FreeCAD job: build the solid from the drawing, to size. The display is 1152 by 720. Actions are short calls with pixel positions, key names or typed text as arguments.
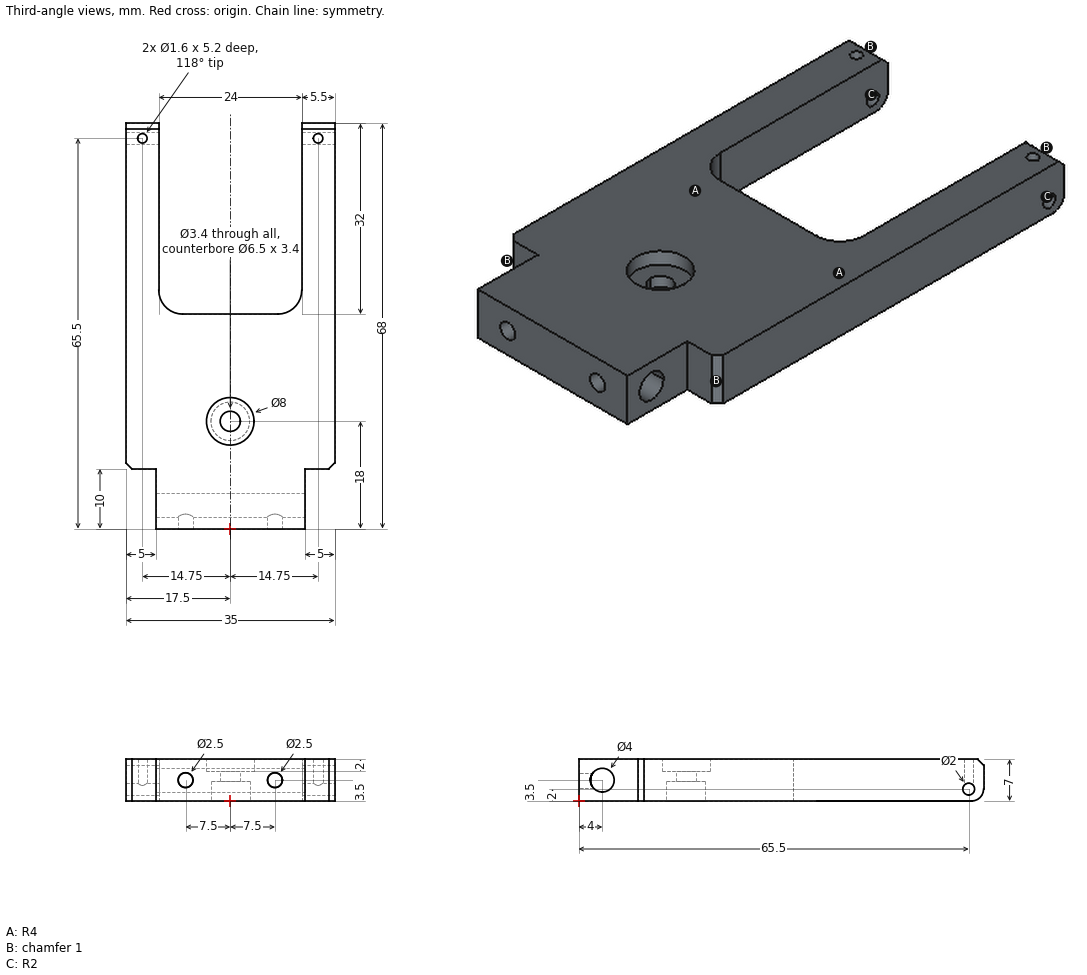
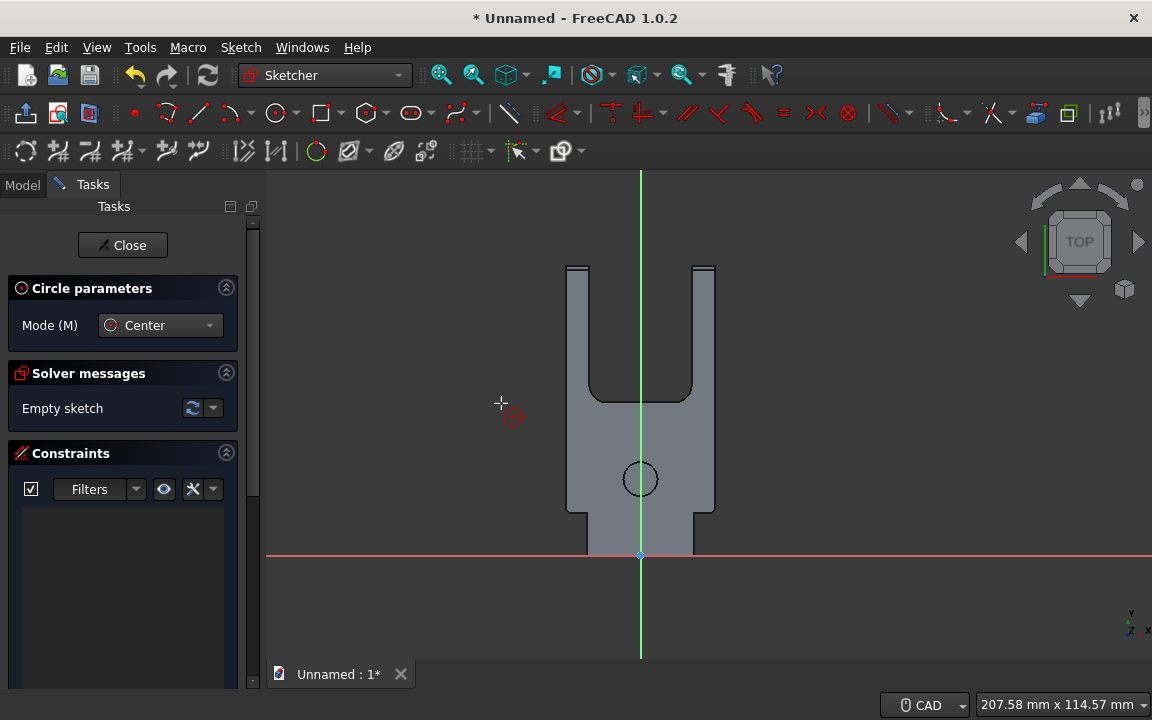
scroll(578, 276, up, 10)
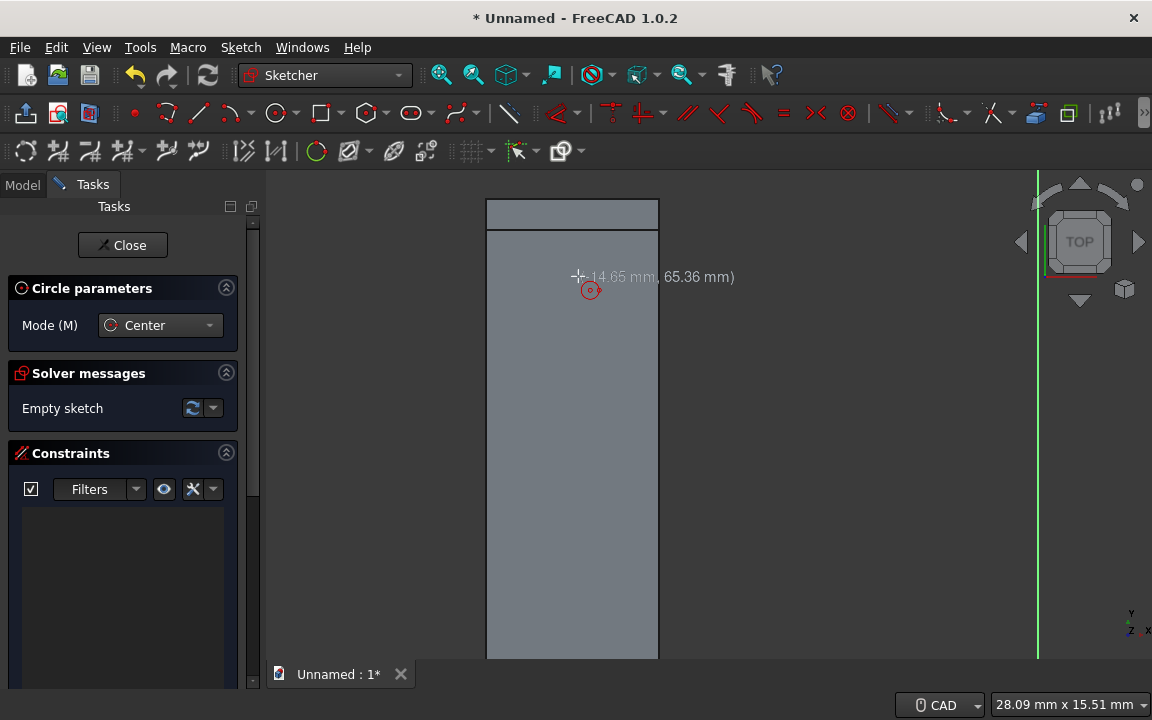
scroll(578, 276, down, 10)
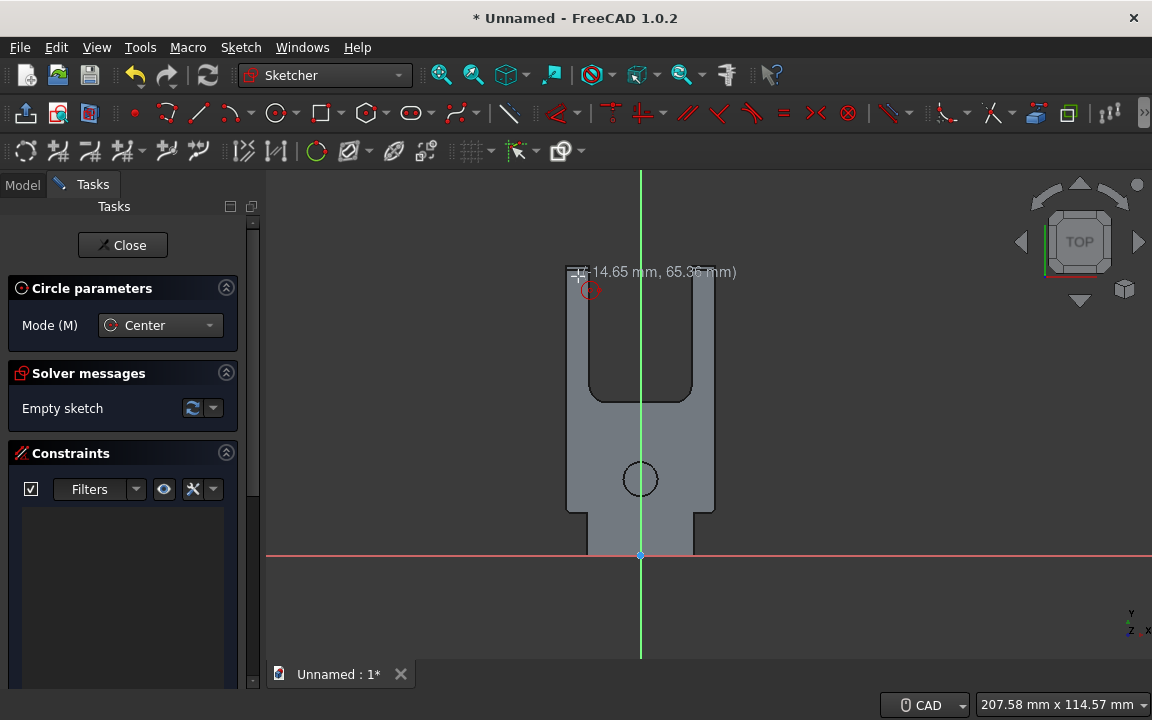
click(578, 276)
move(580, 274)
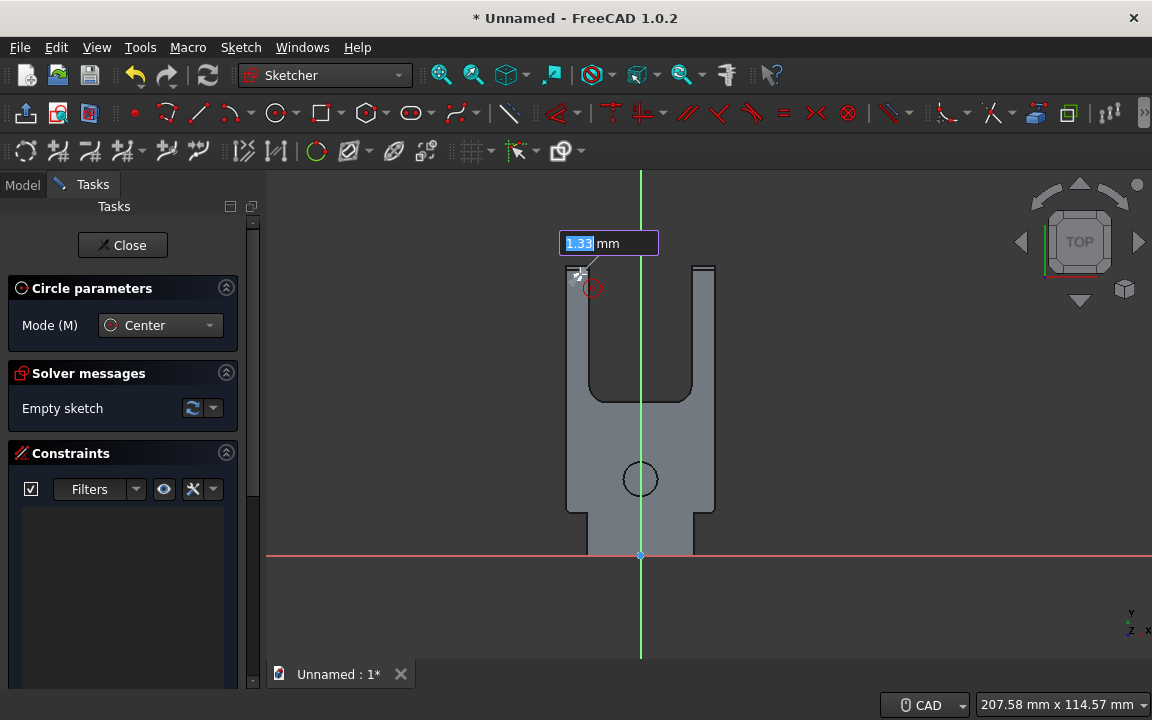
text(1.6)
key(Return)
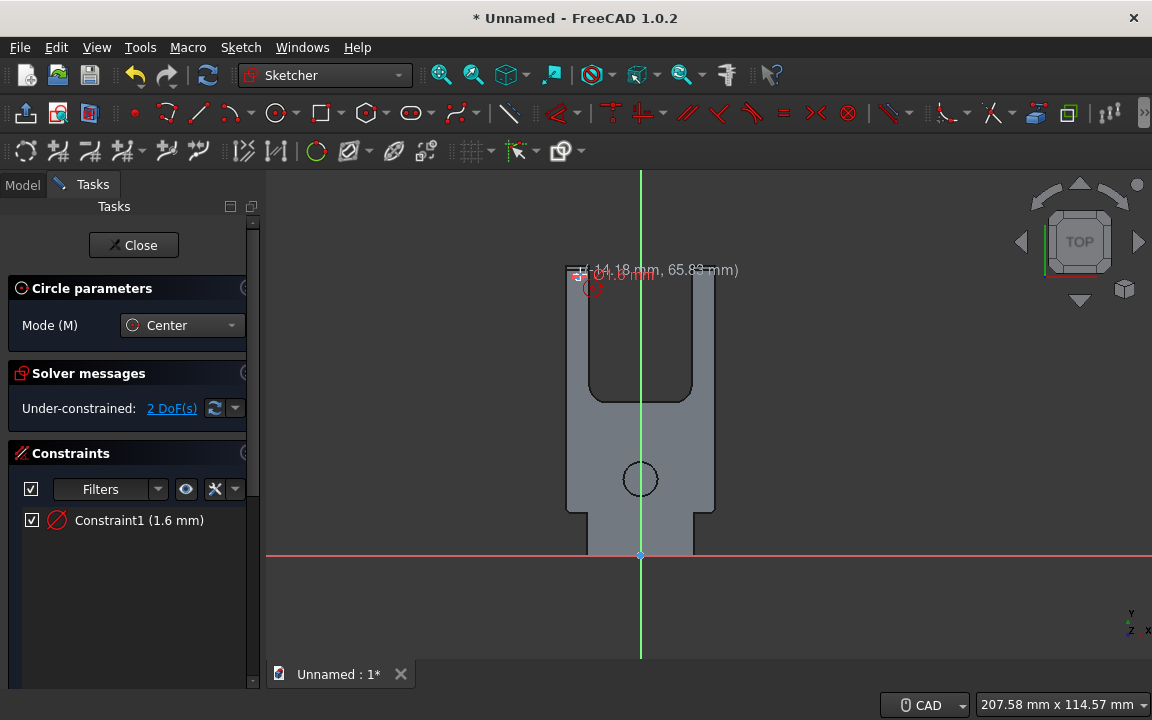
scroll(703, 276, up, 10)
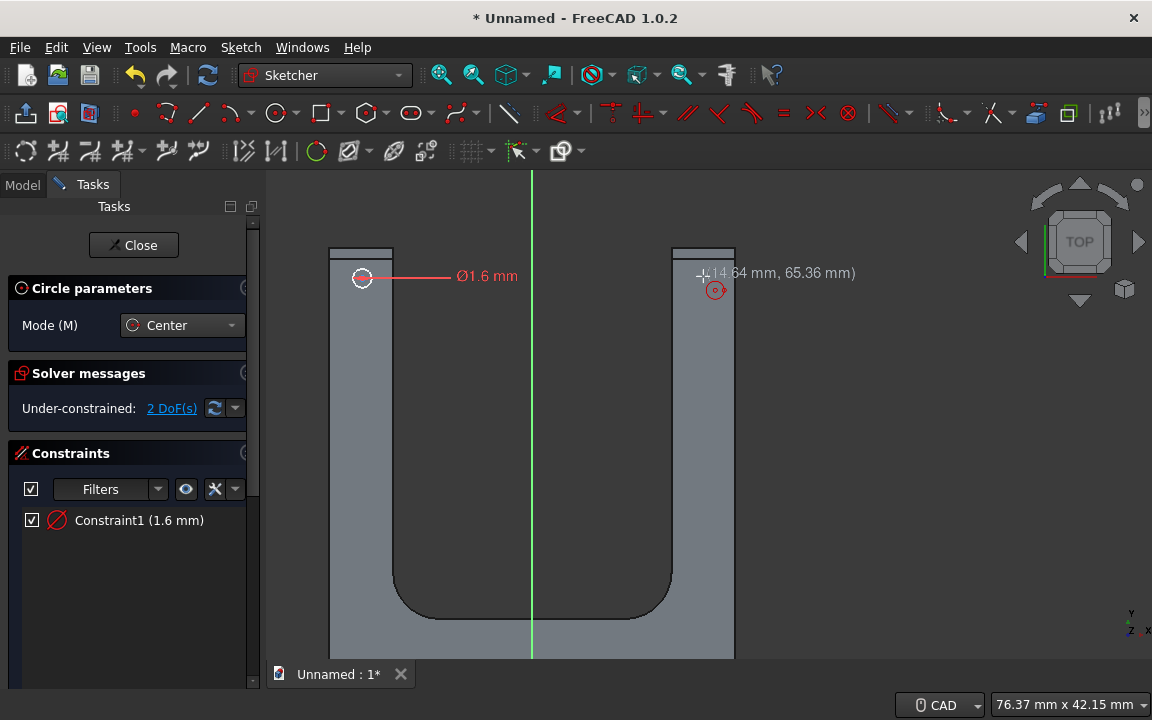
scroll(703, 276, down, 10)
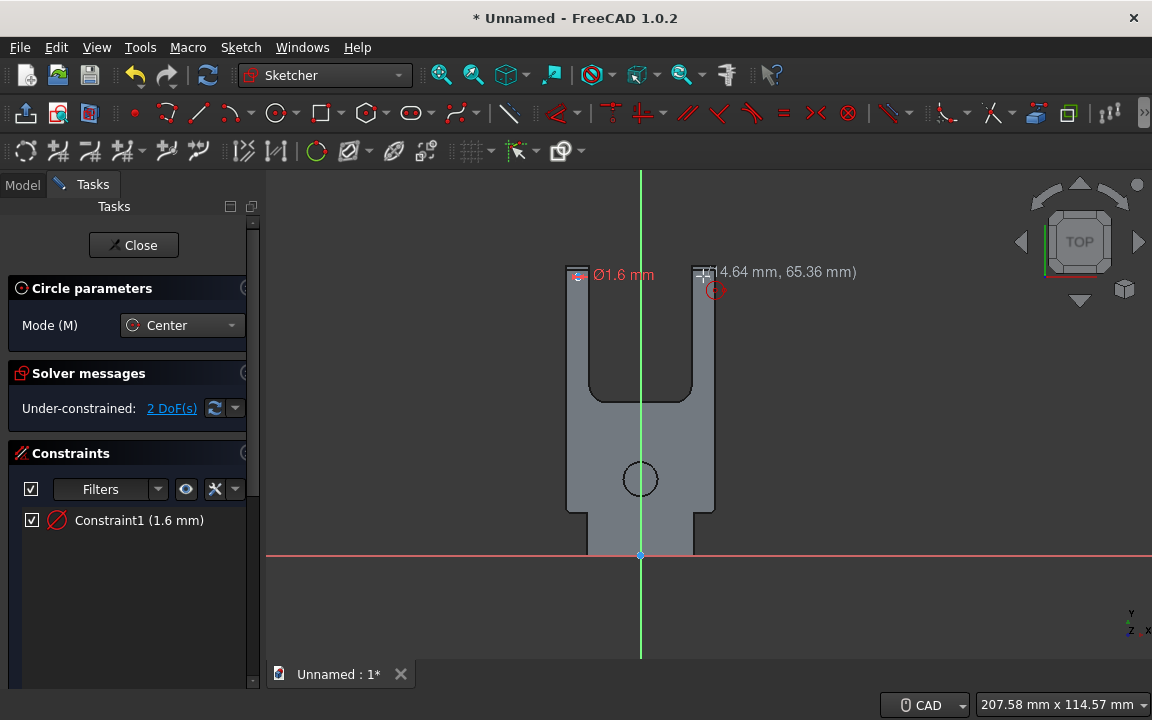
click(703, 276)
move(706, 274)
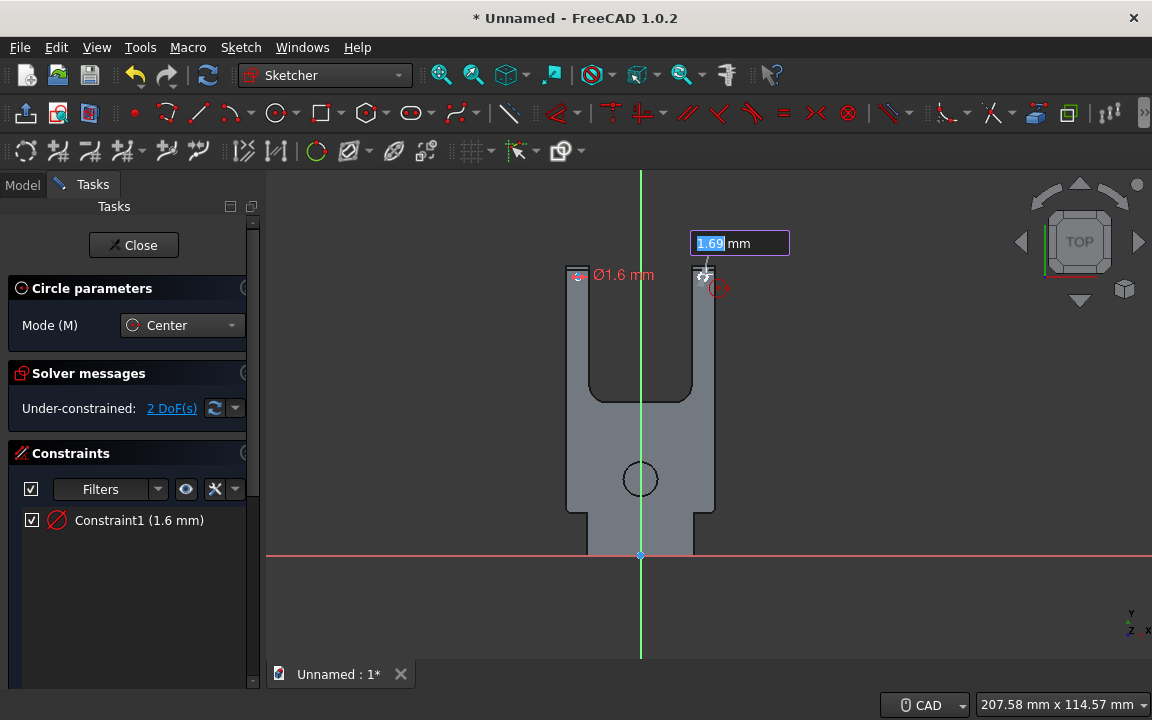
text(1.6)
key(Return)
key(Escape)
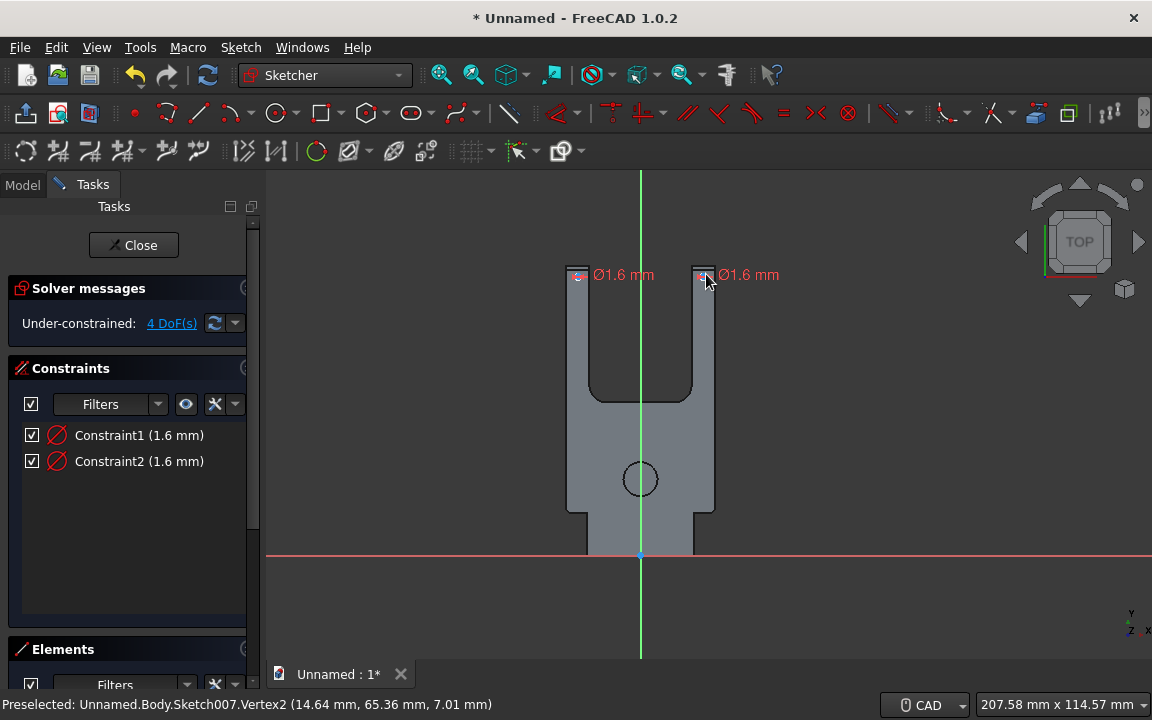
click(578, 277)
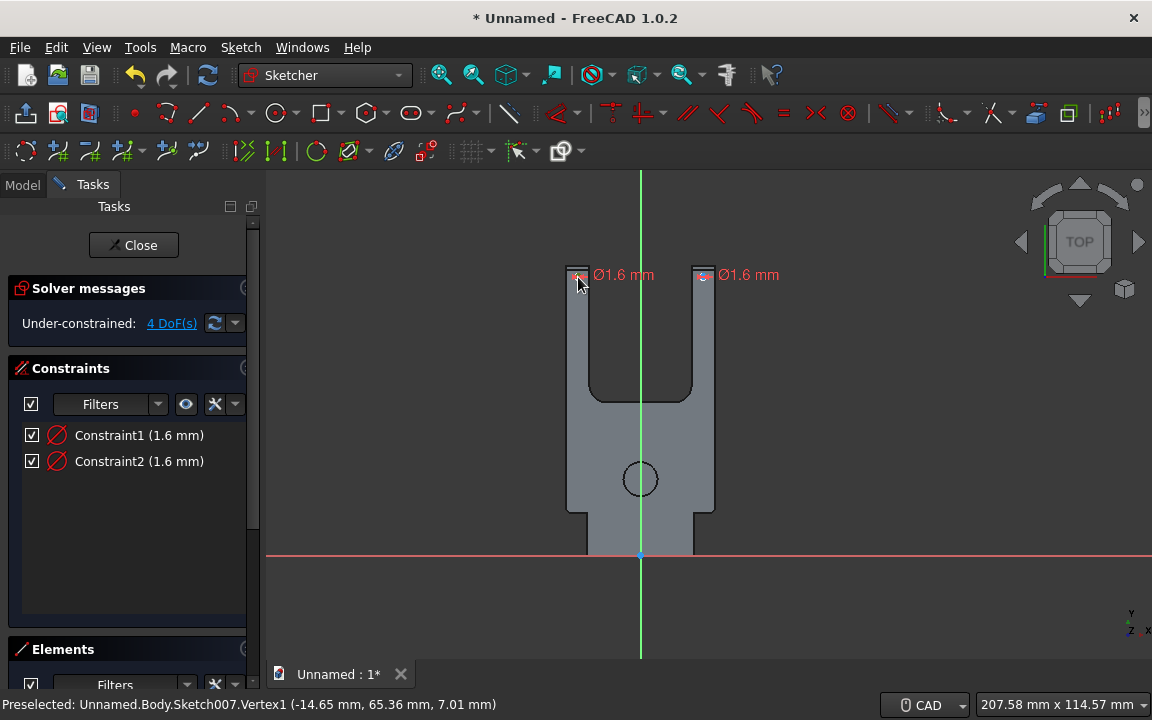
click(703, 277)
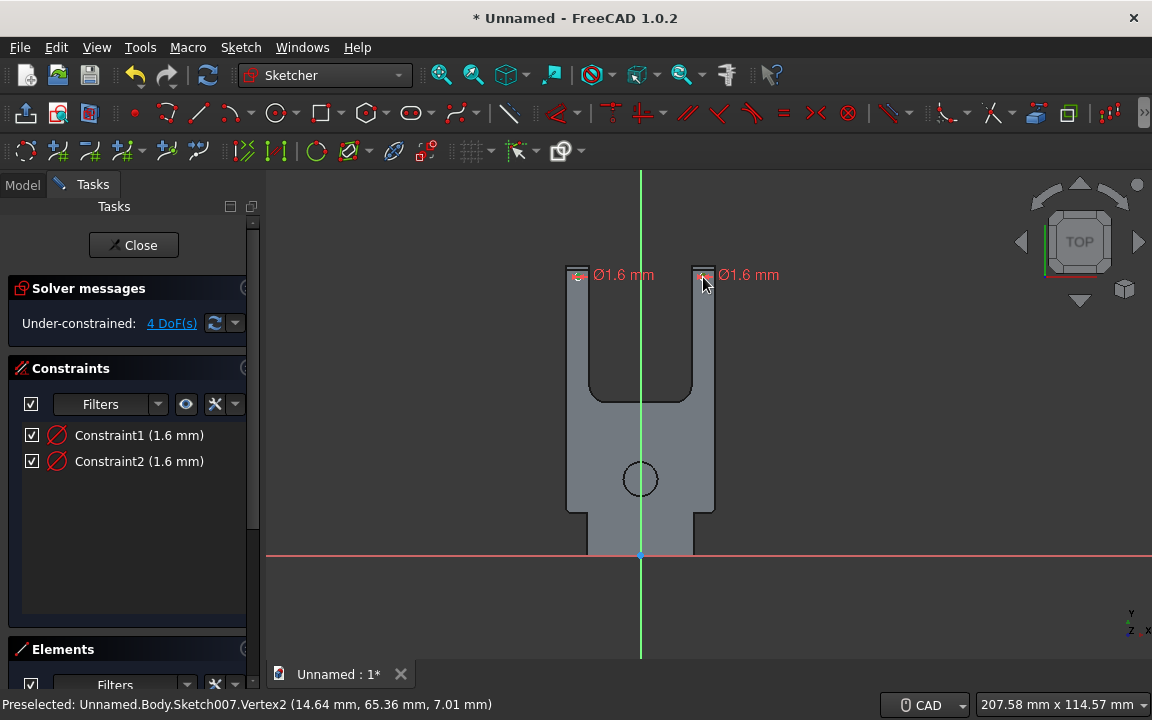
key(h)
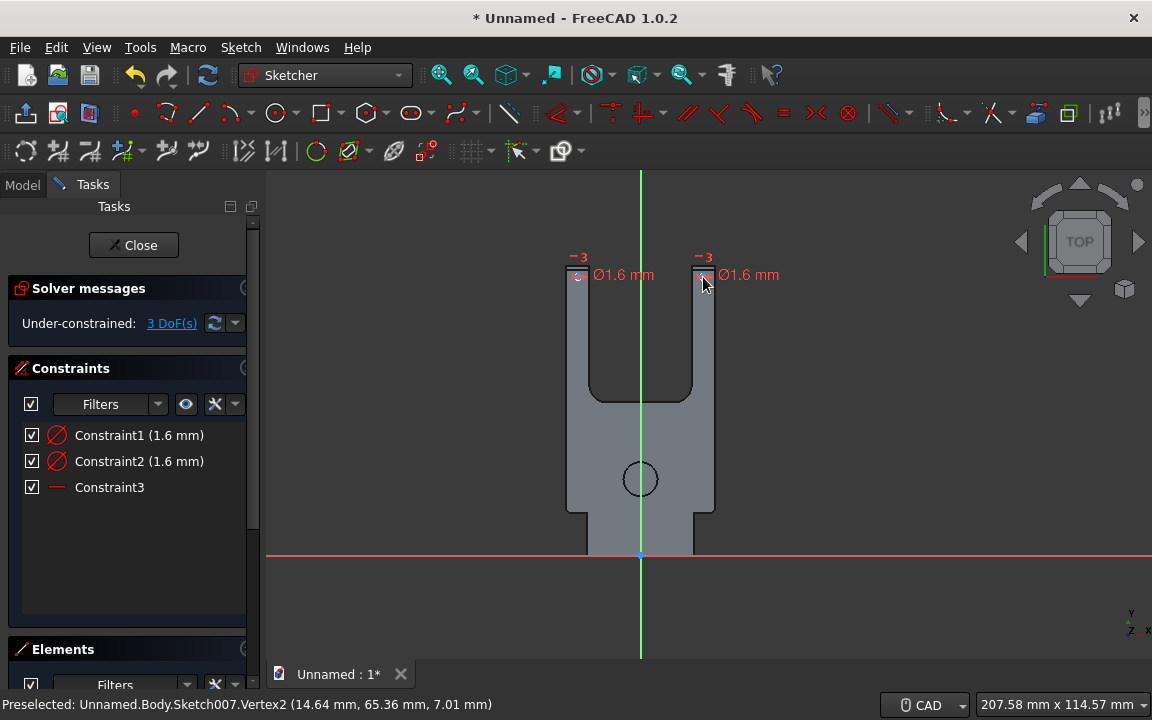
key(d)